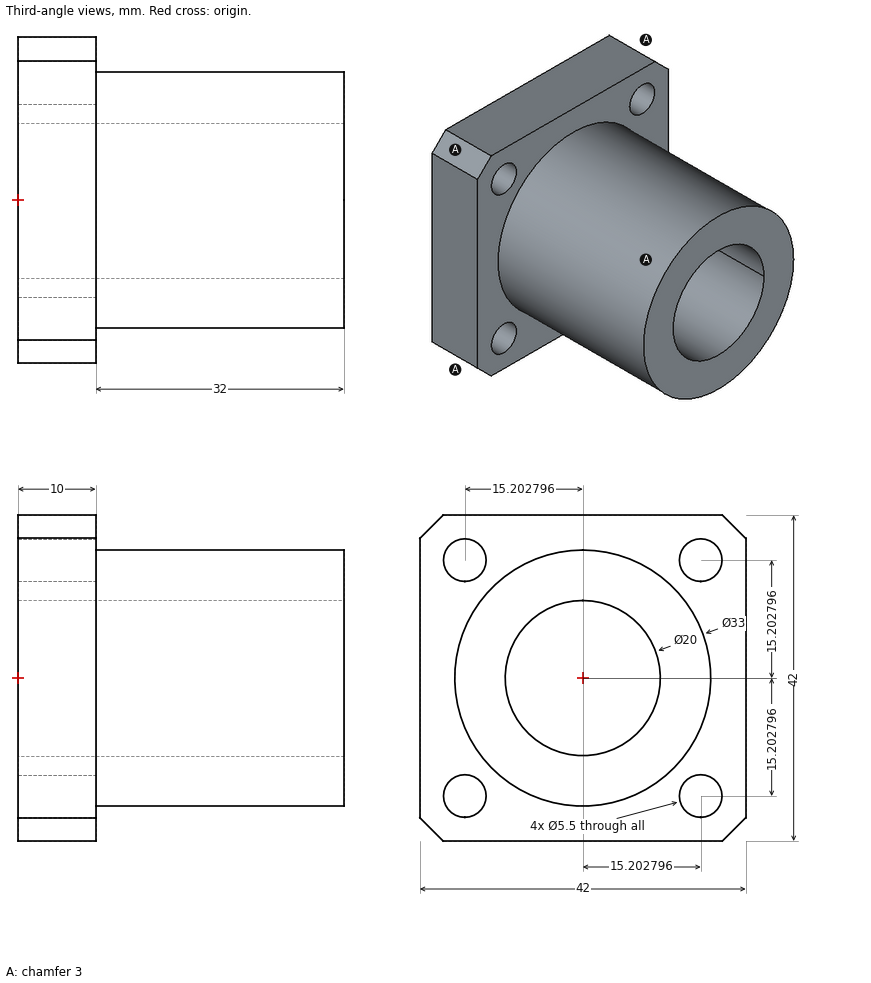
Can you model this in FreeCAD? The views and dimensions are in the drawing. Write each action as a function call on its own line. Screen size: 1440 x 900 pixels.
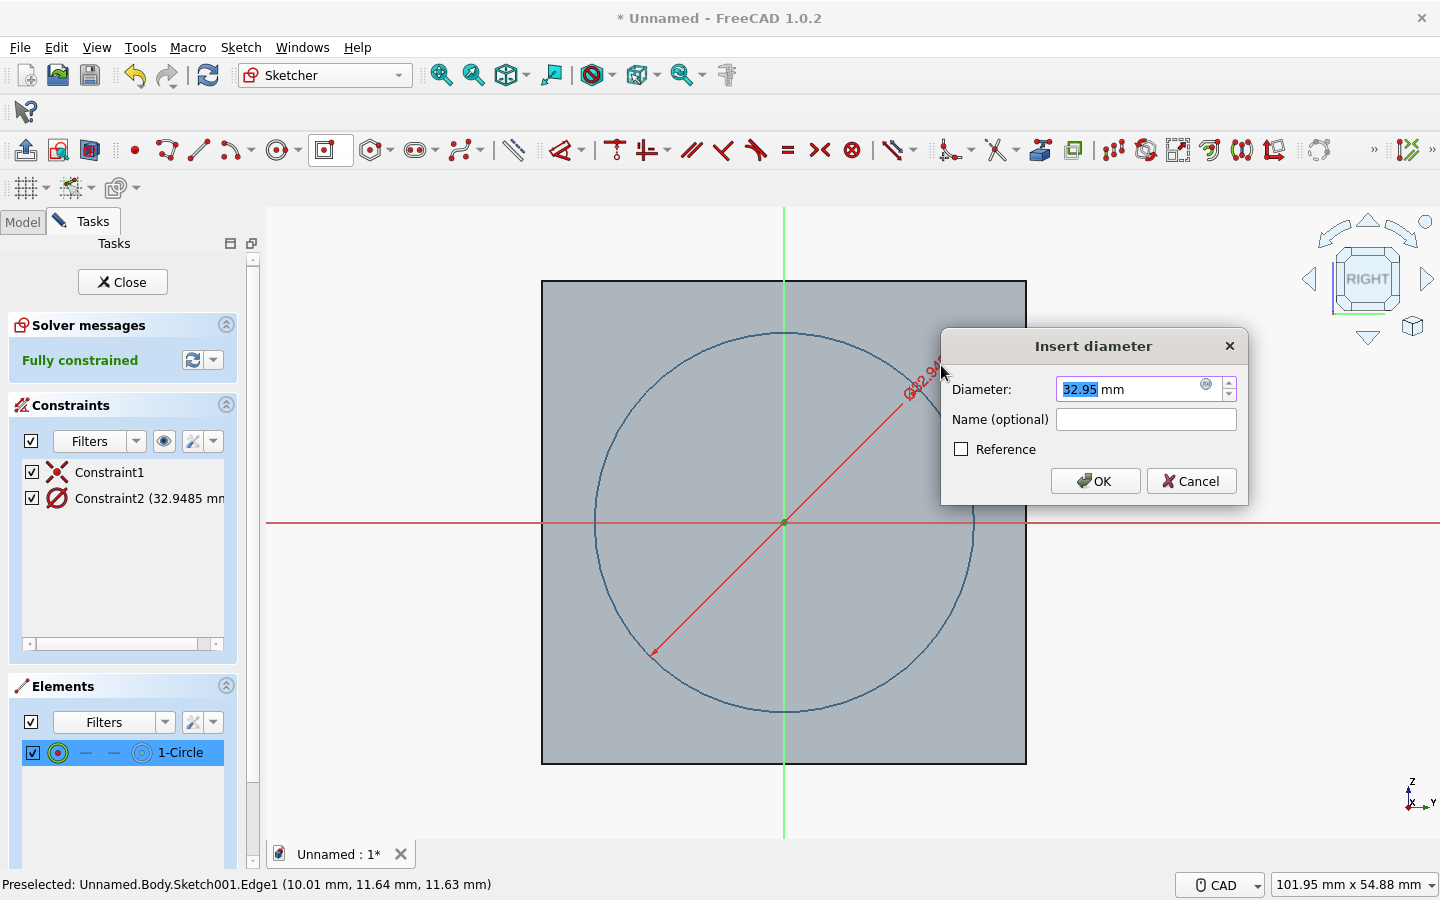
text(33)
key(Return)
key(Escape)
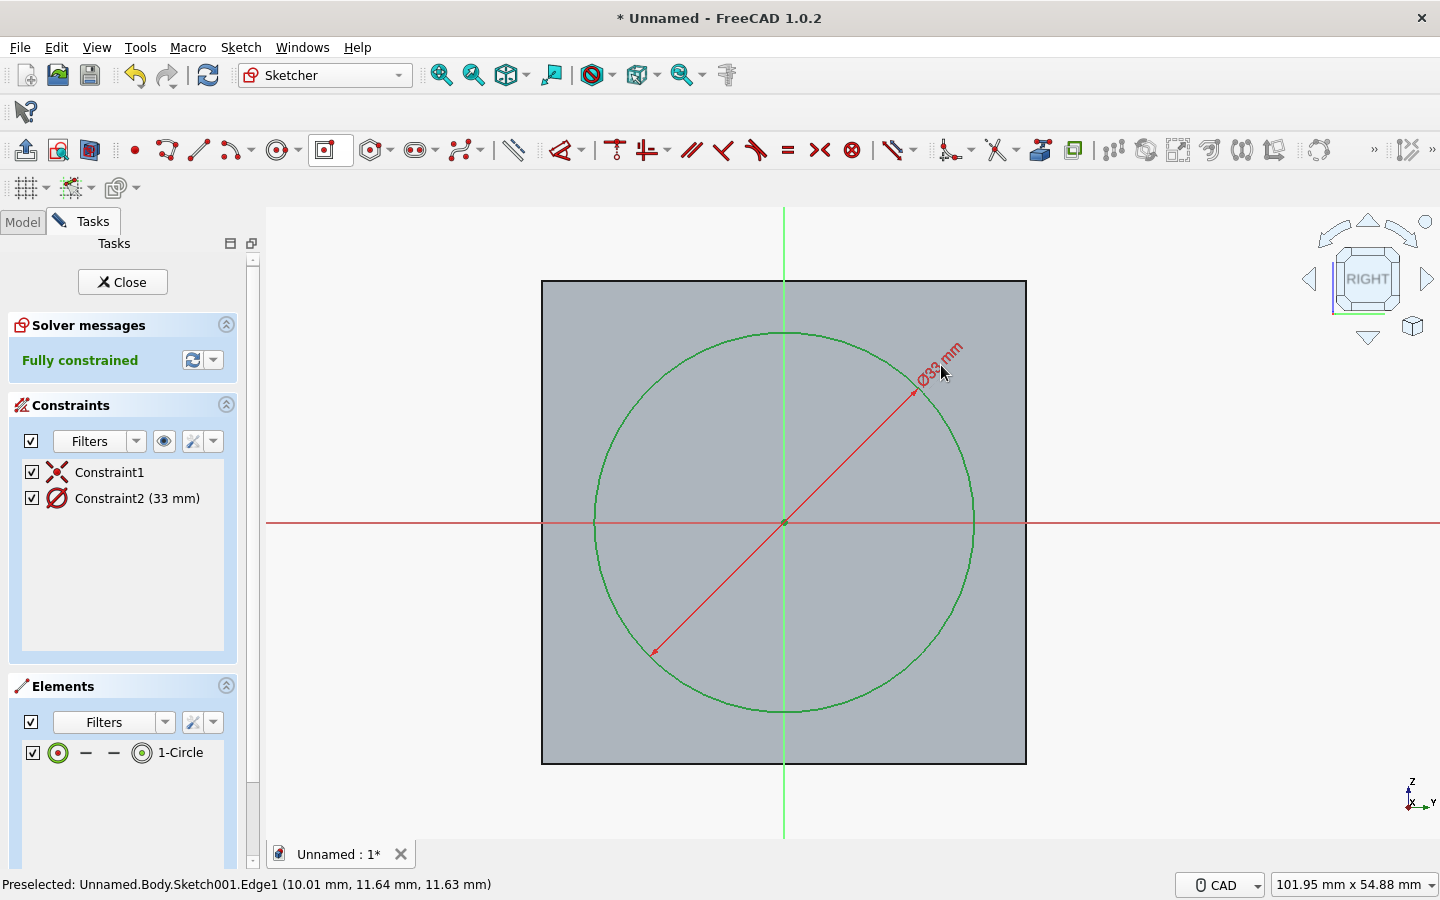
click(123, 282)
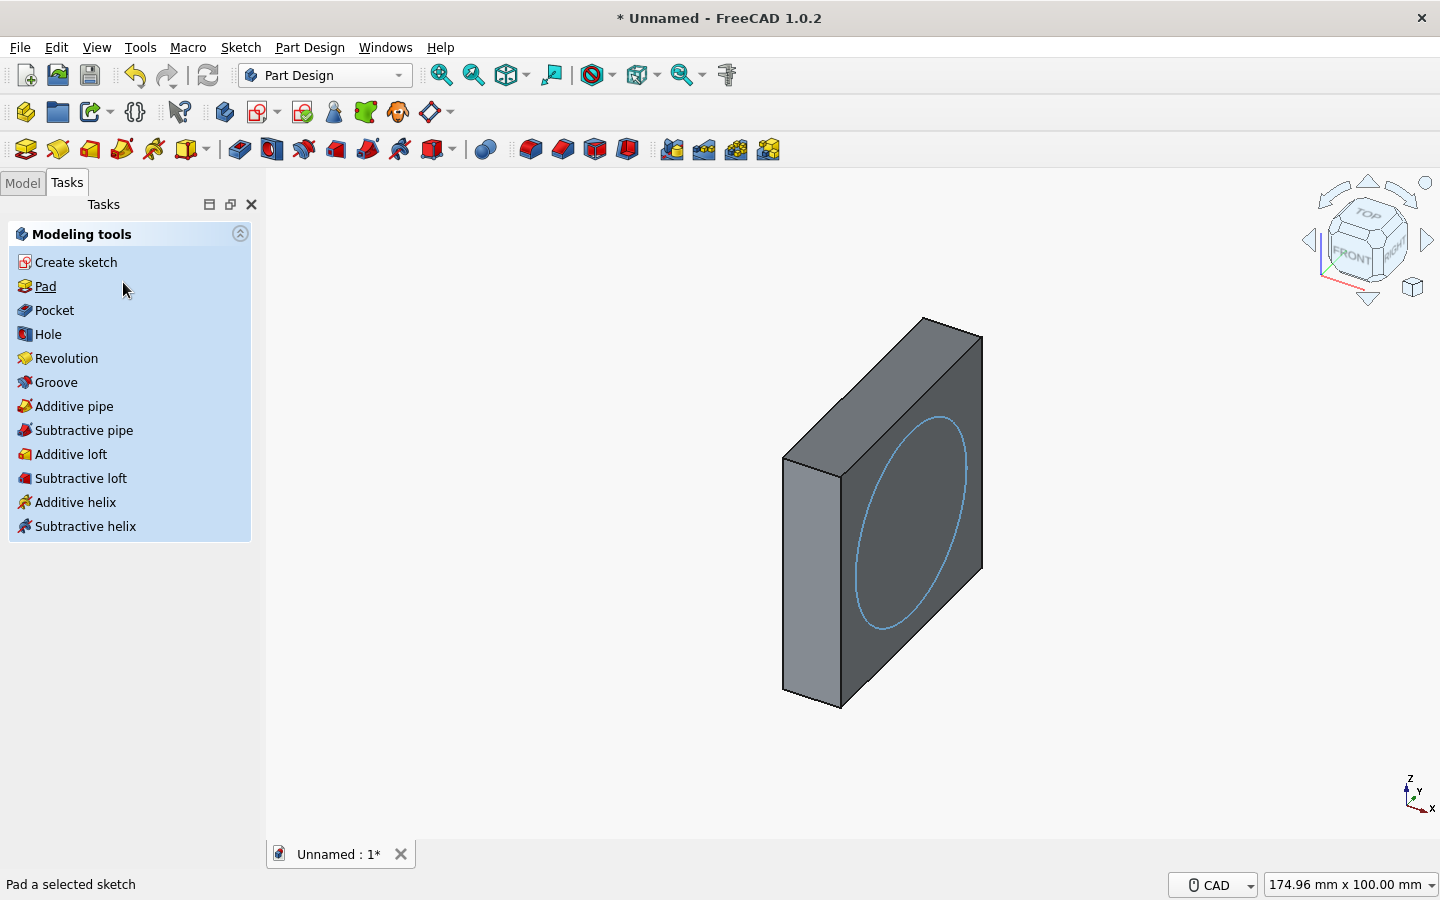
click(26, 150)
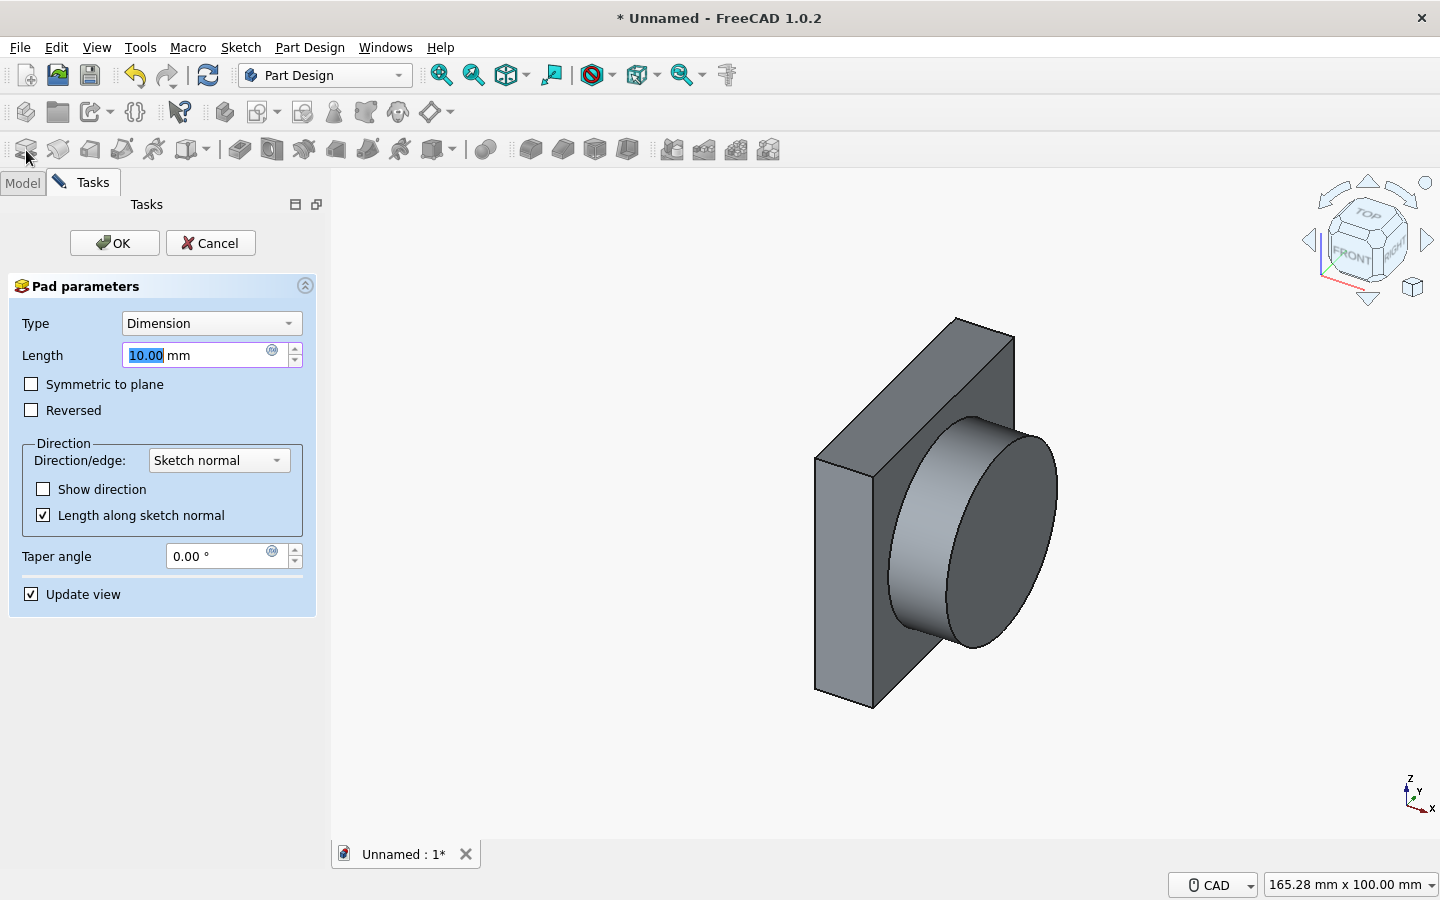
text(32)
key(Tab)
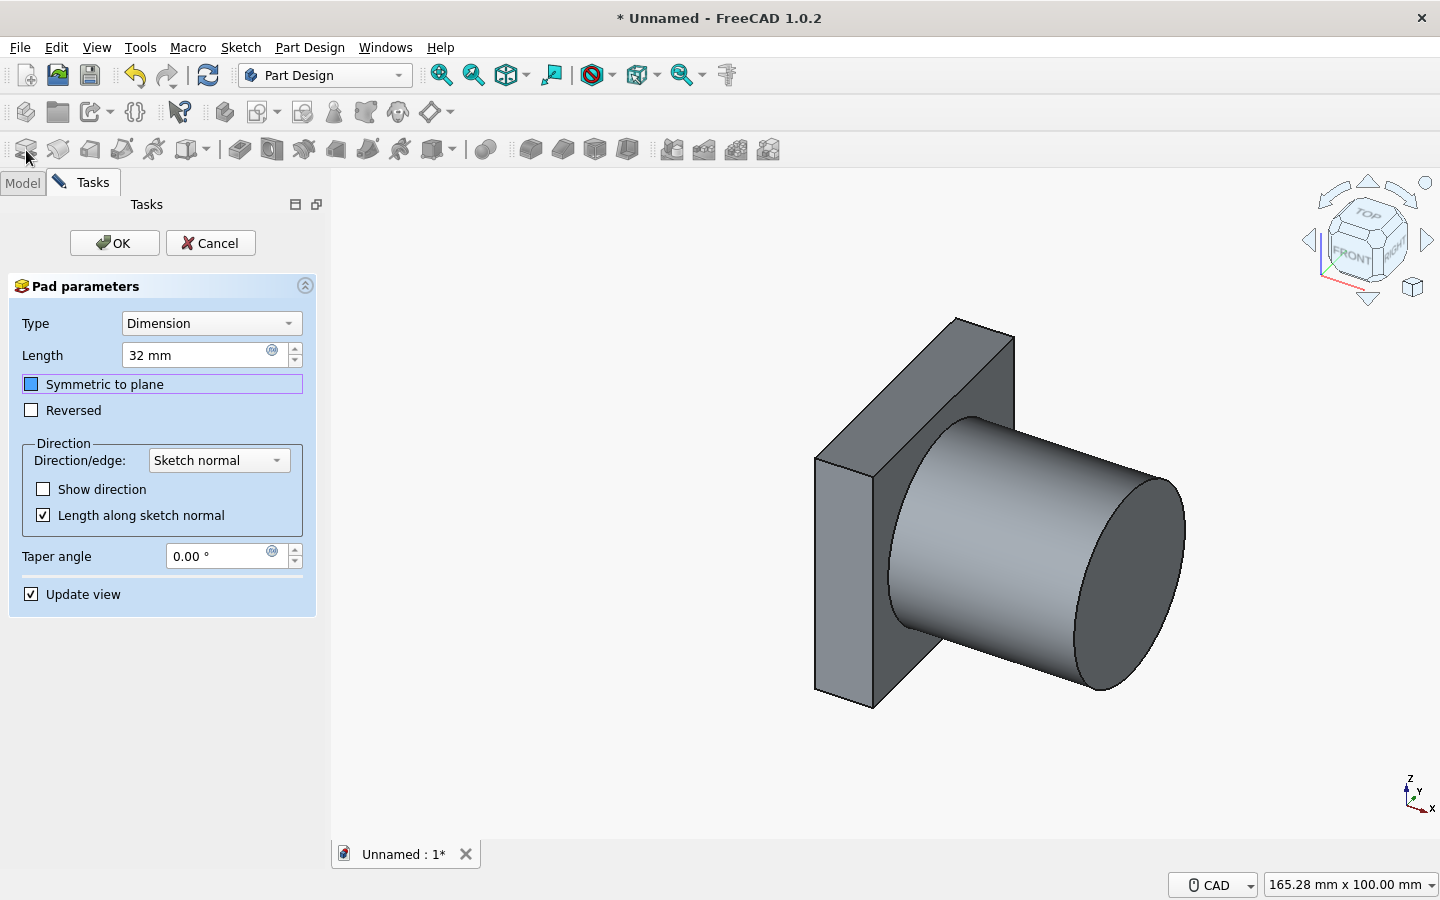
click(115, 243)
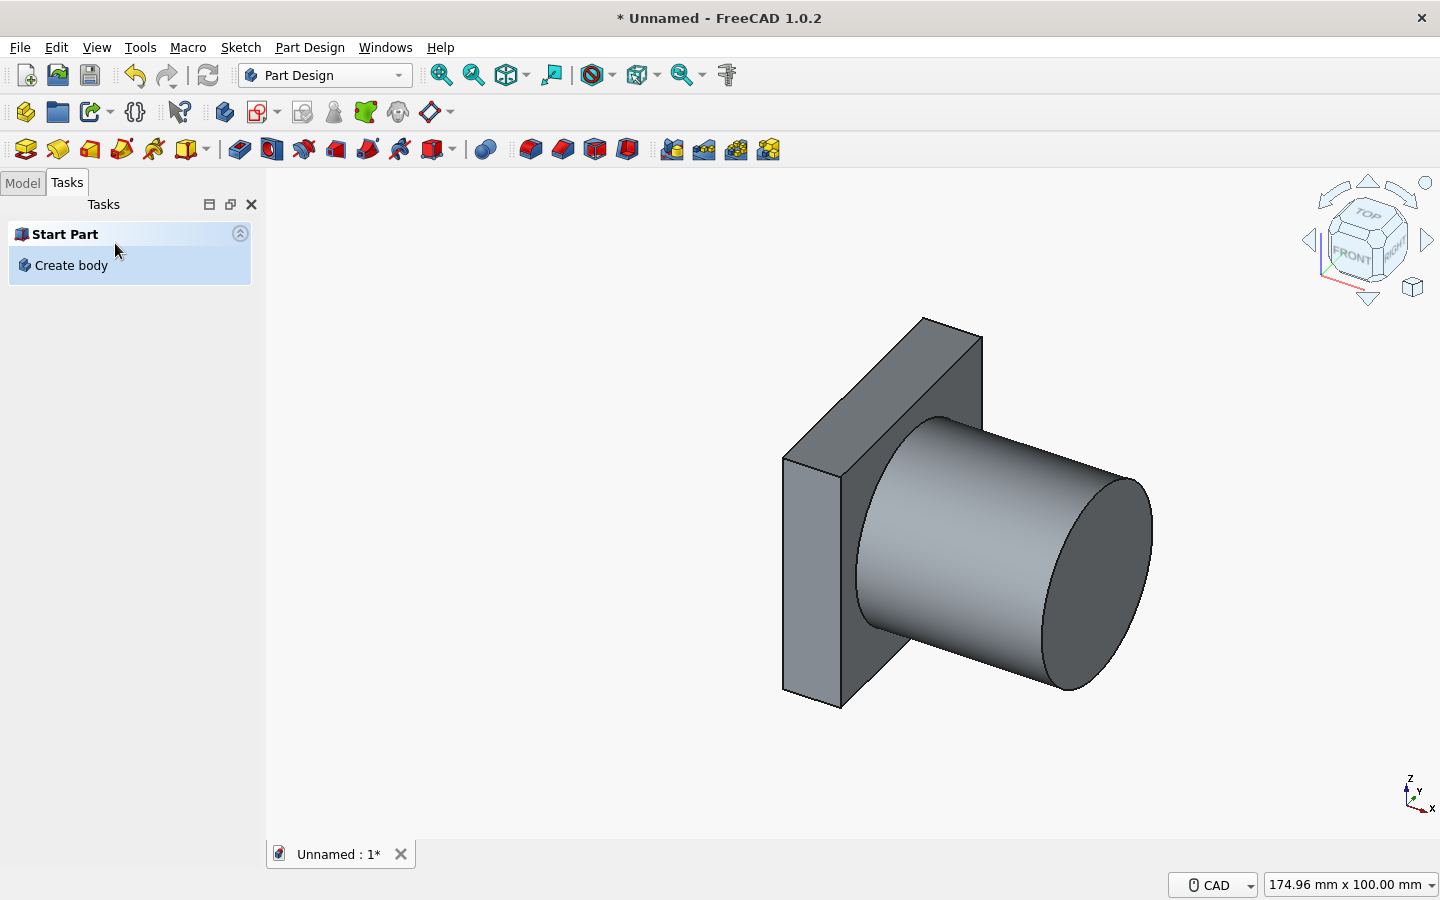
click(258, 112)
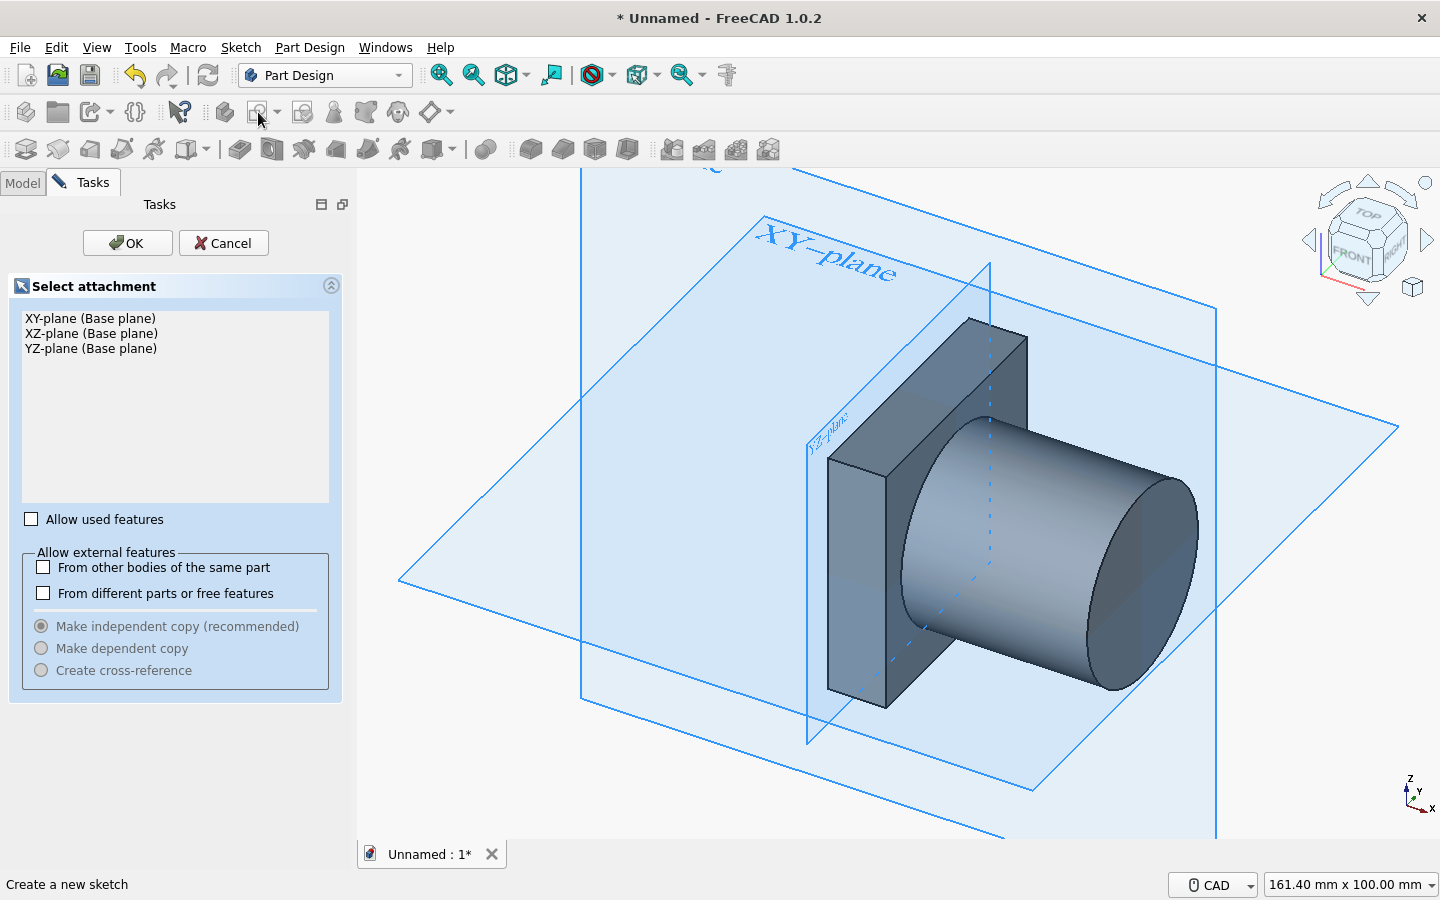
click(82, 348)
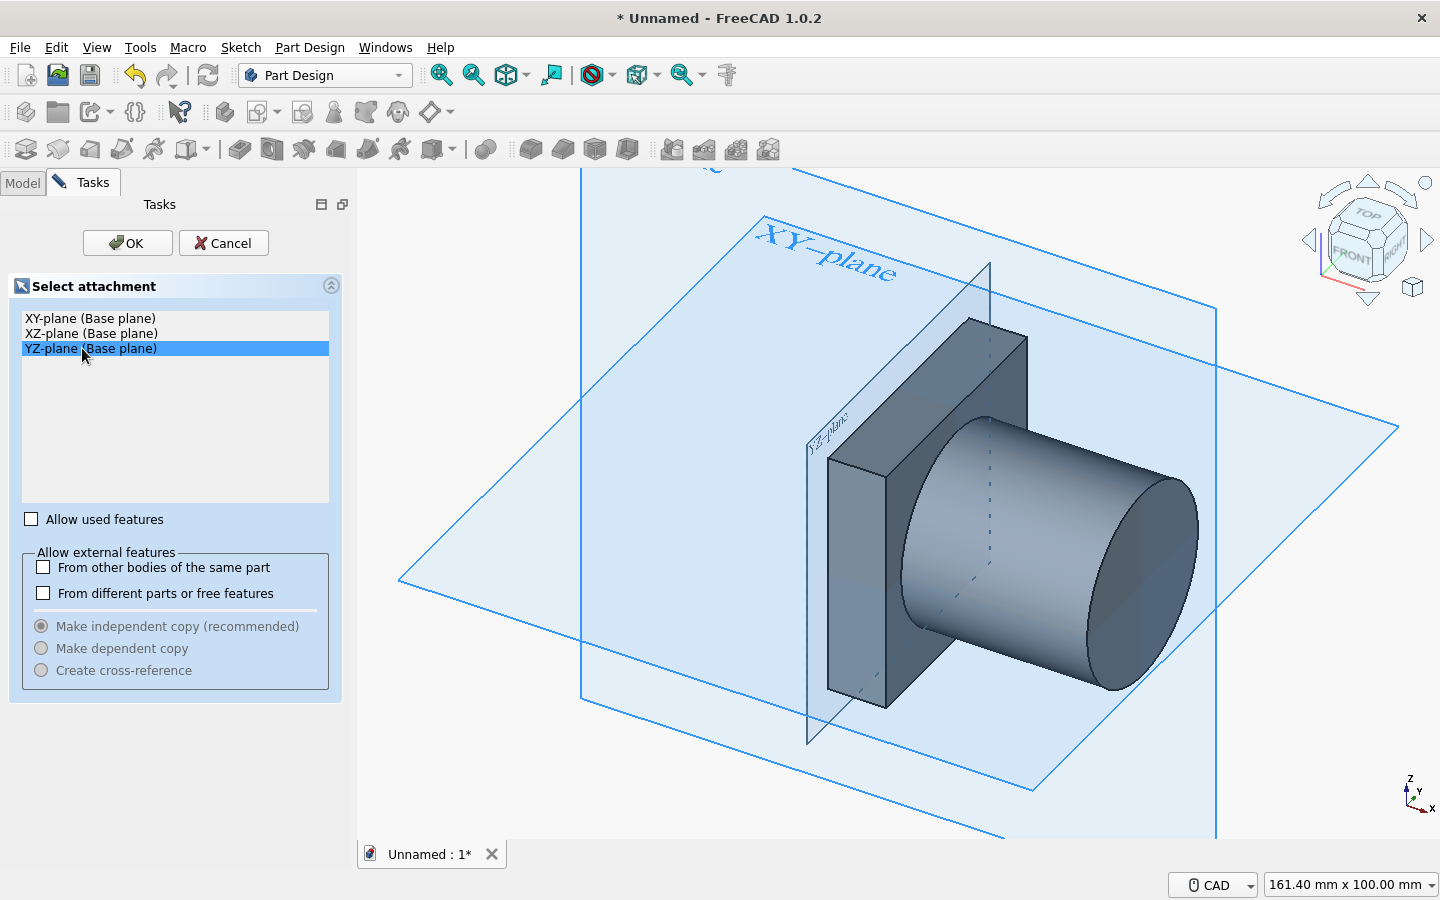
click(128, 243)